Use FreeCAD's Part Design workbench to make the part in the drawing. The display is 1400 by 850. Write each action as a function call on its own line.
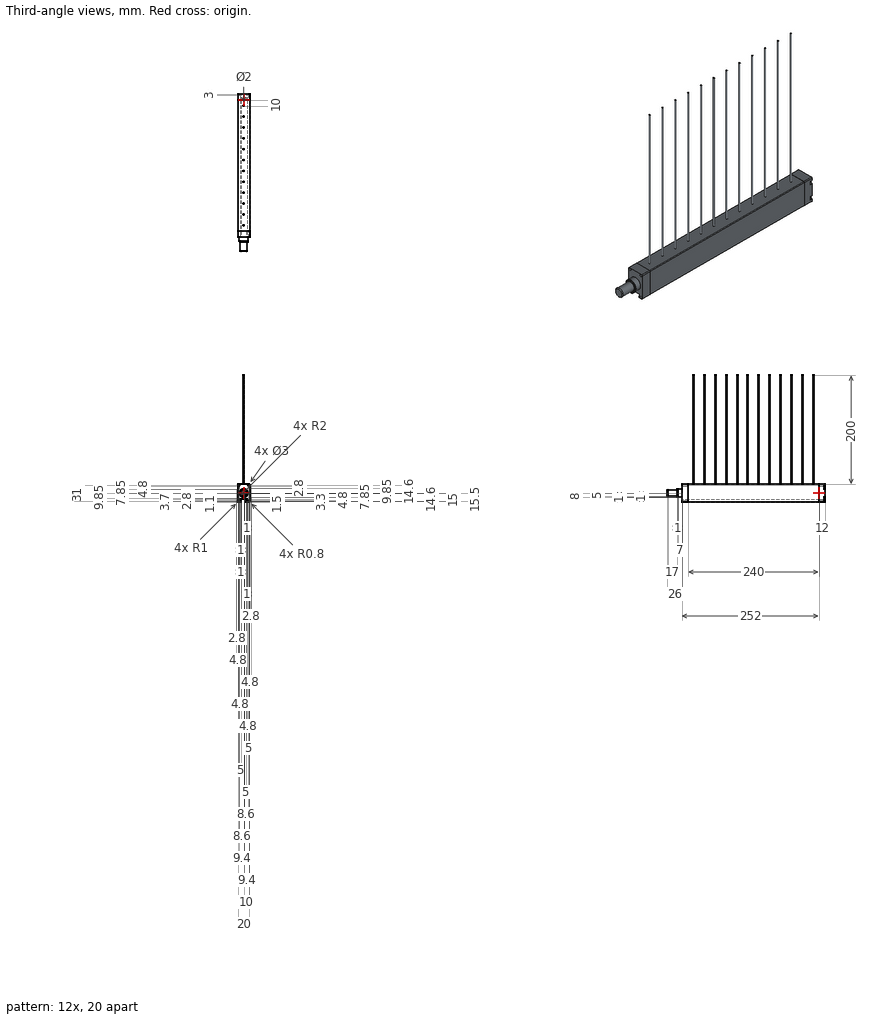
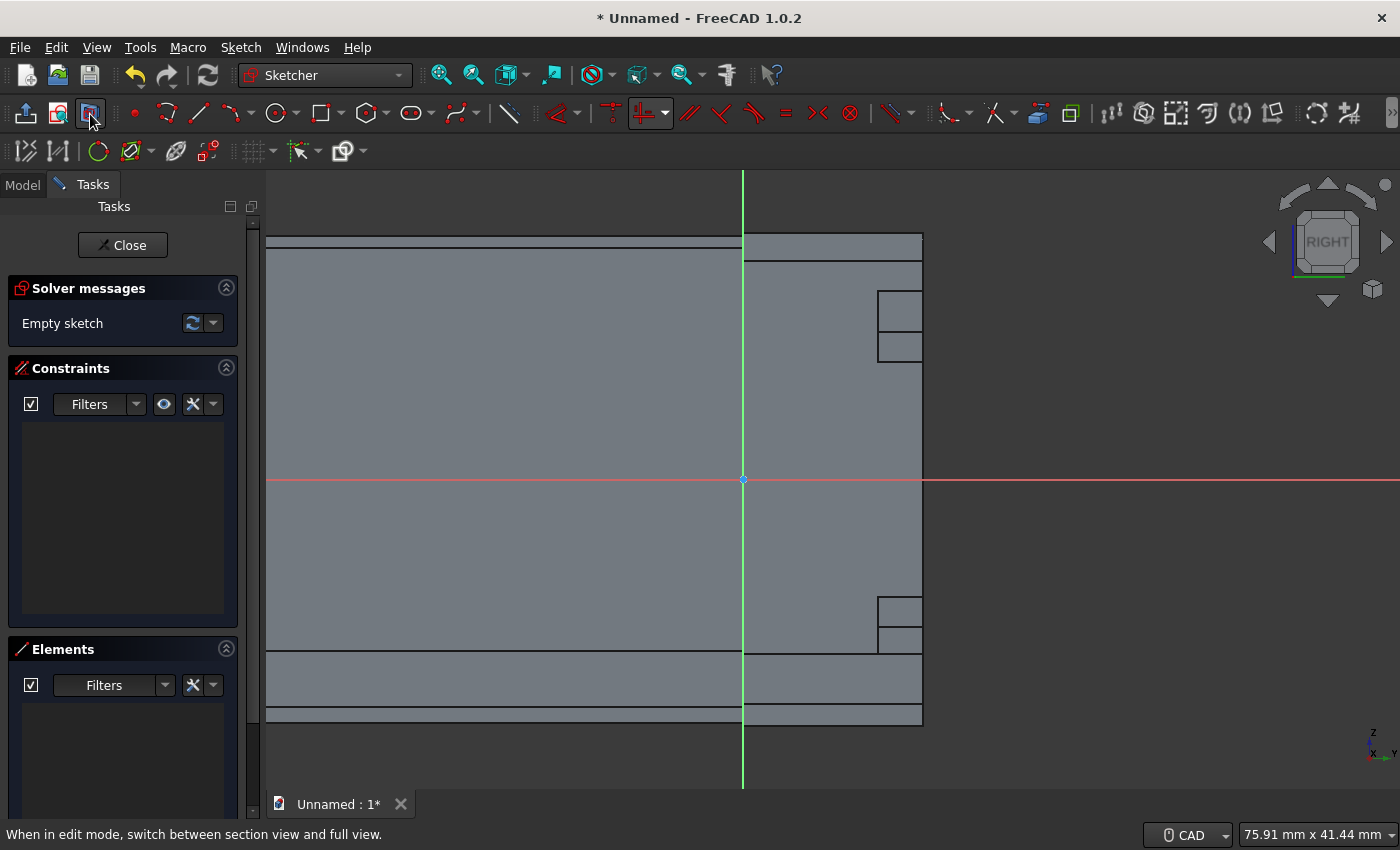
scroll(764, 480, down, 5)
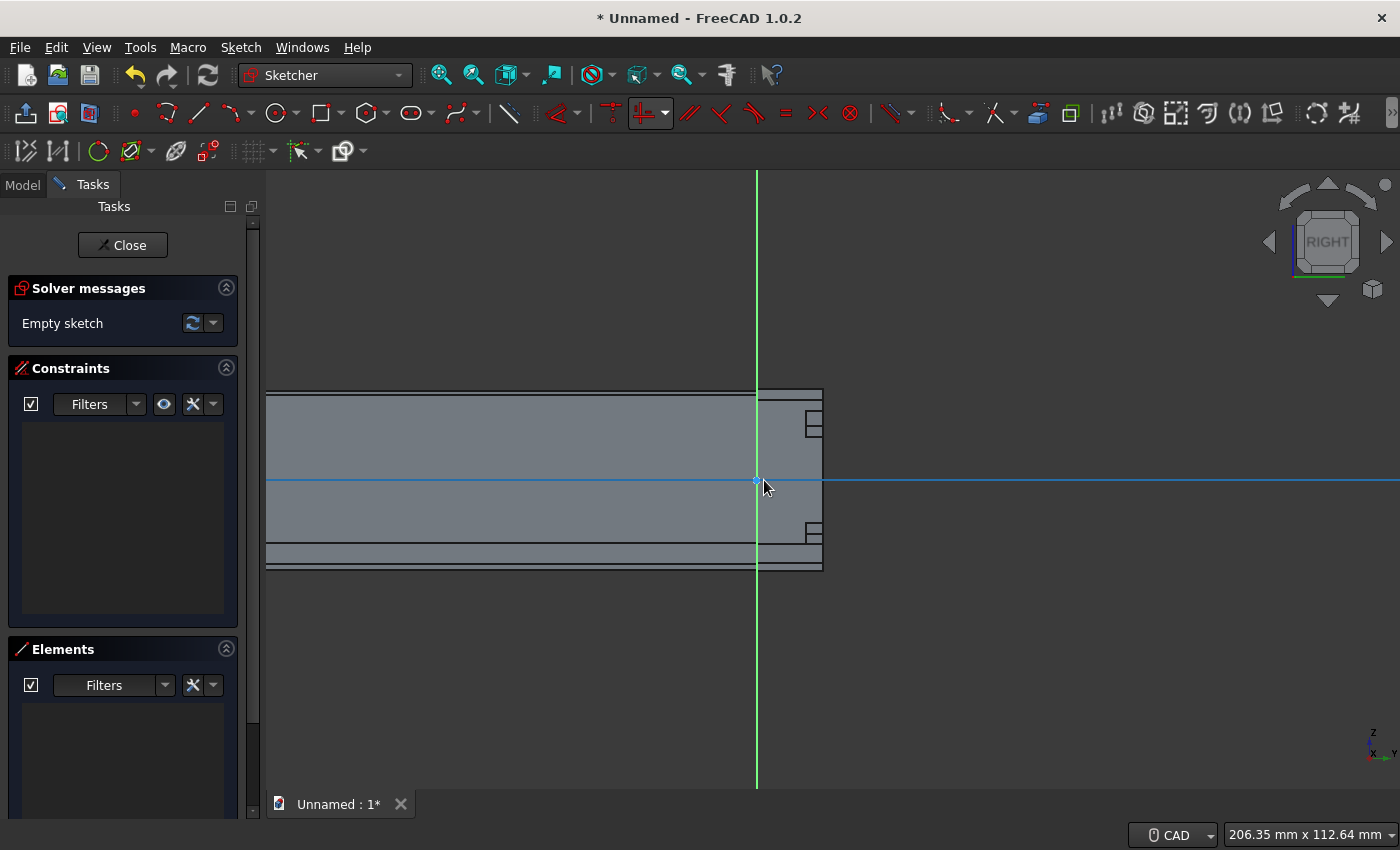
scroll(764, 480, down, 5)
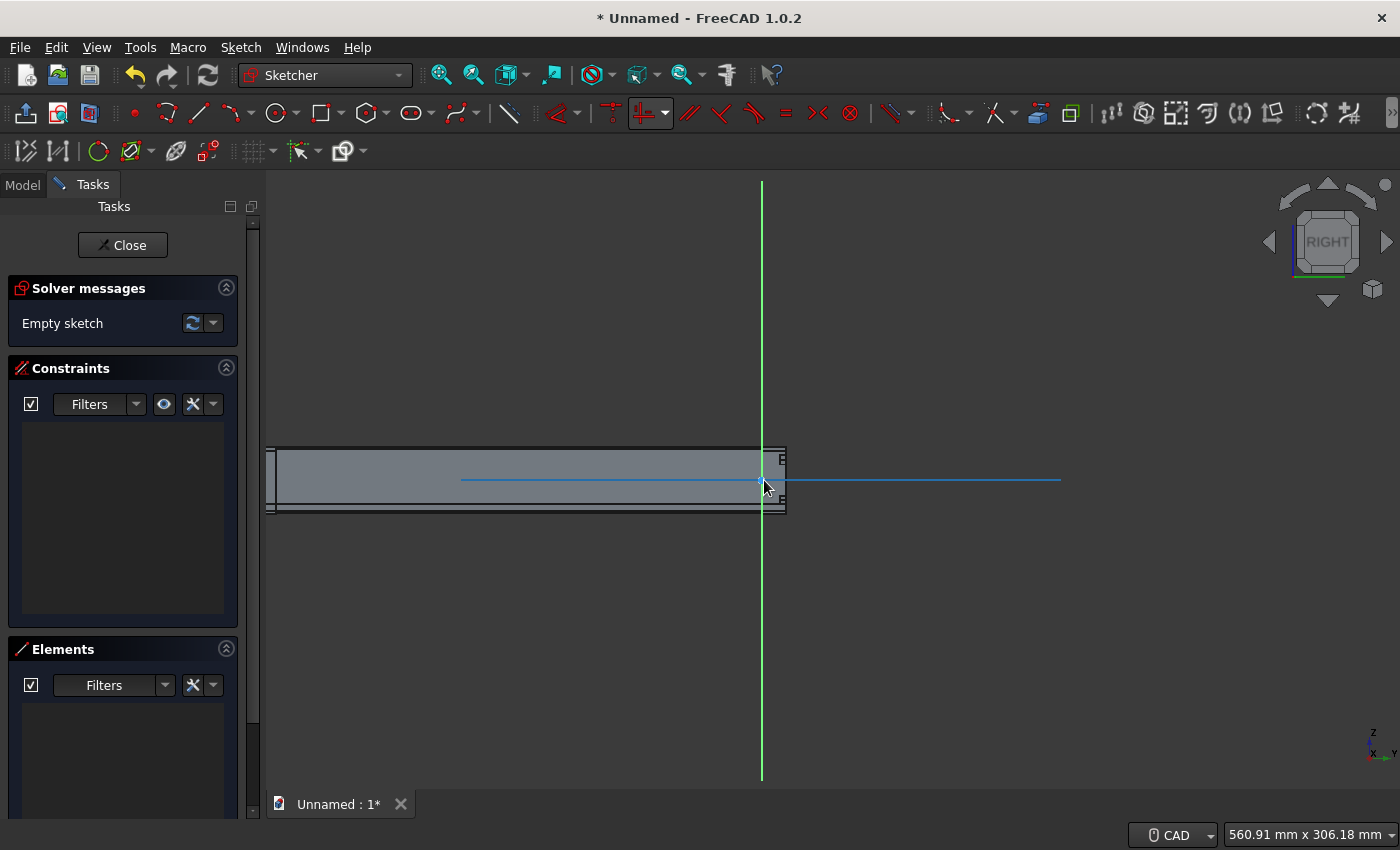
scroll(764, 480, down, 5)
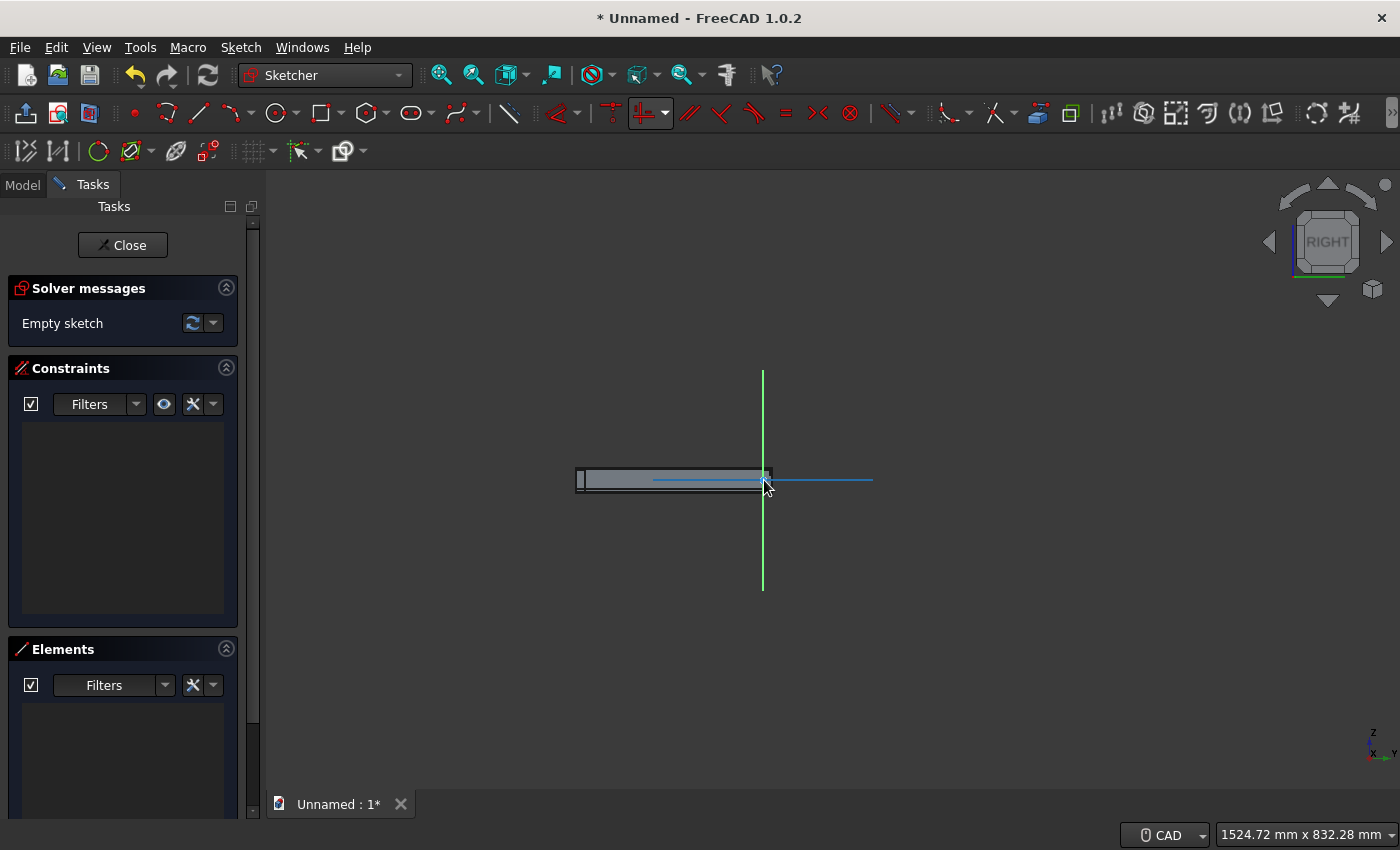
scroll(556, 484, up, 15)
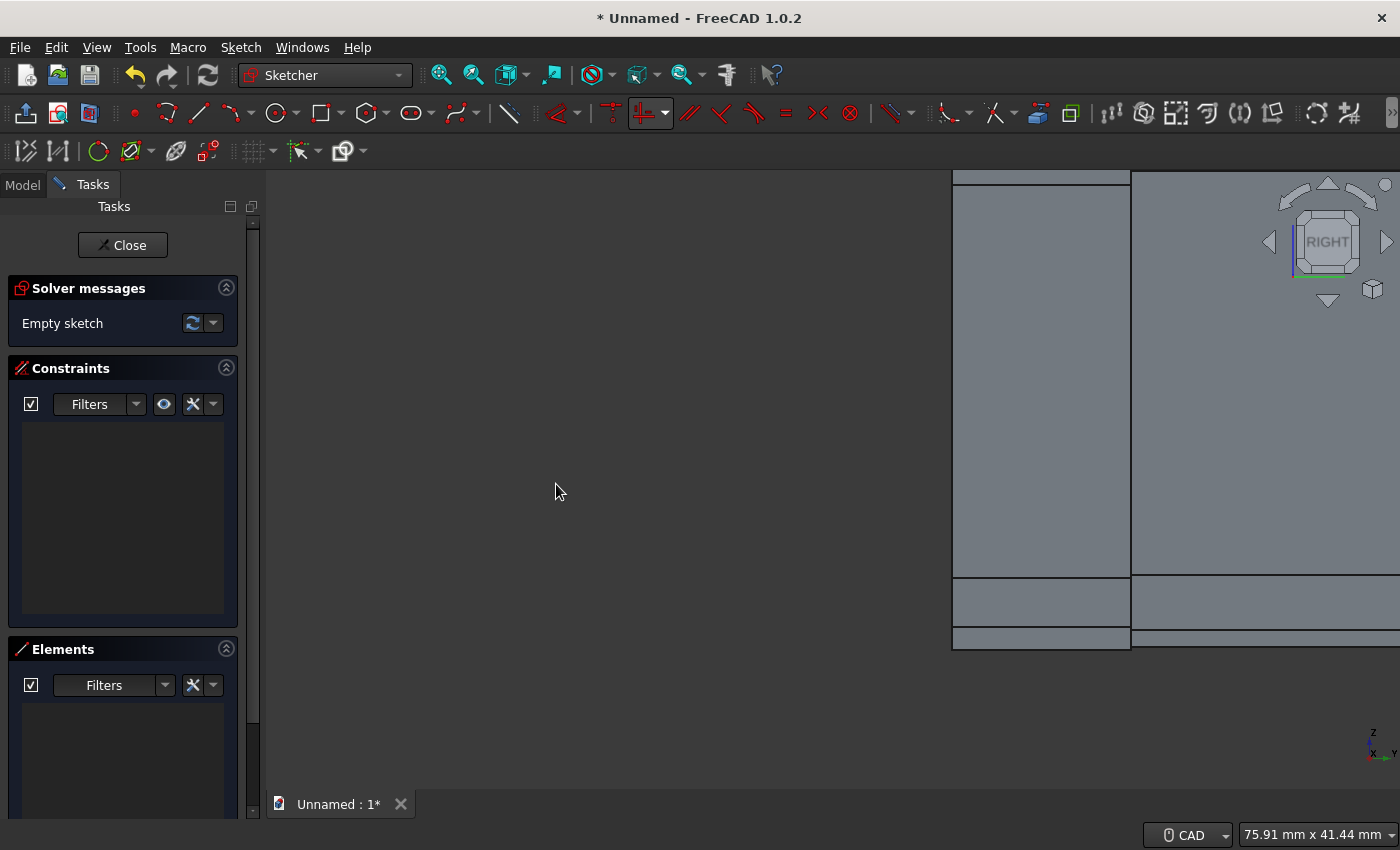
scroll(750, 442, up, 3)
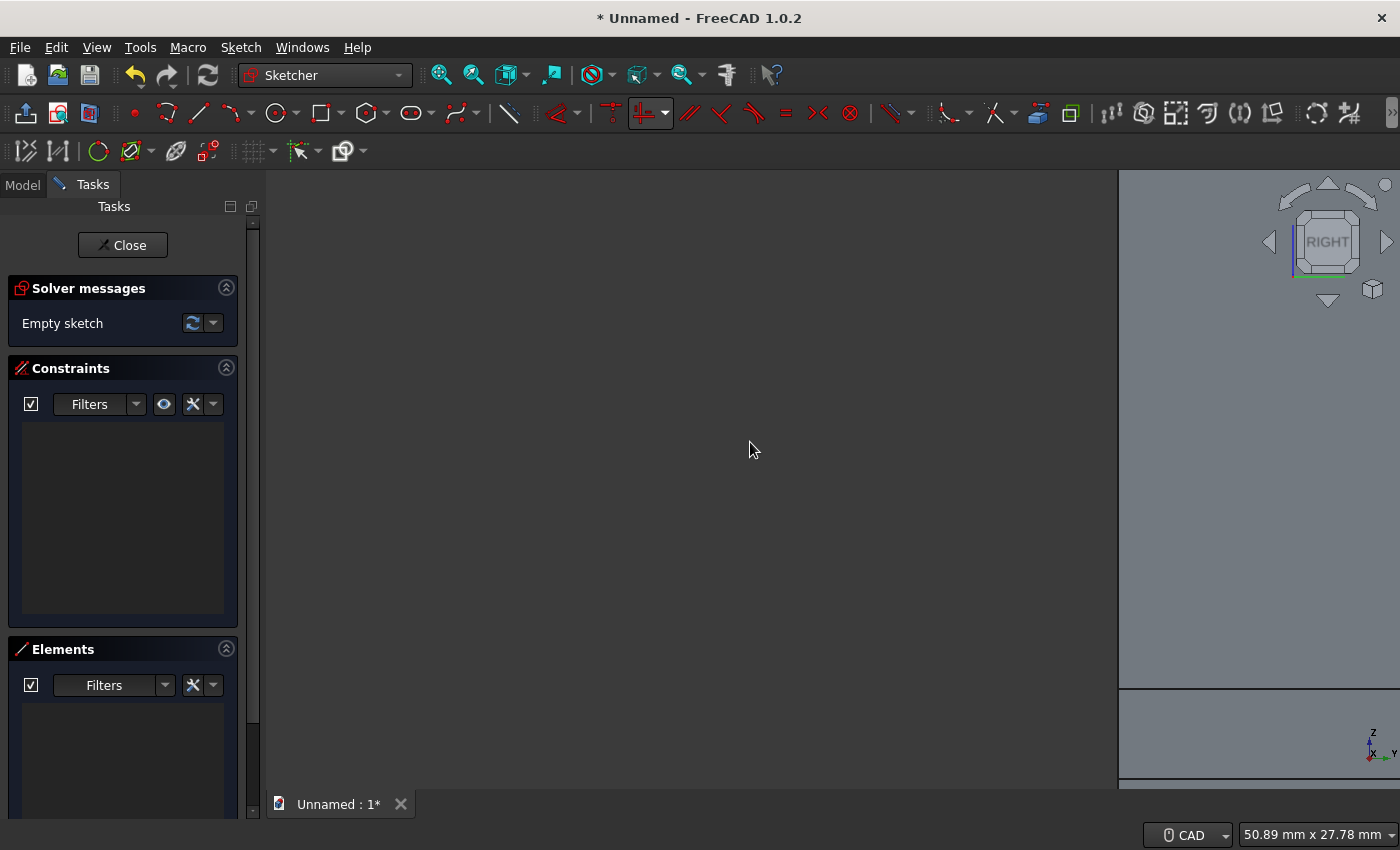
click(168, 114)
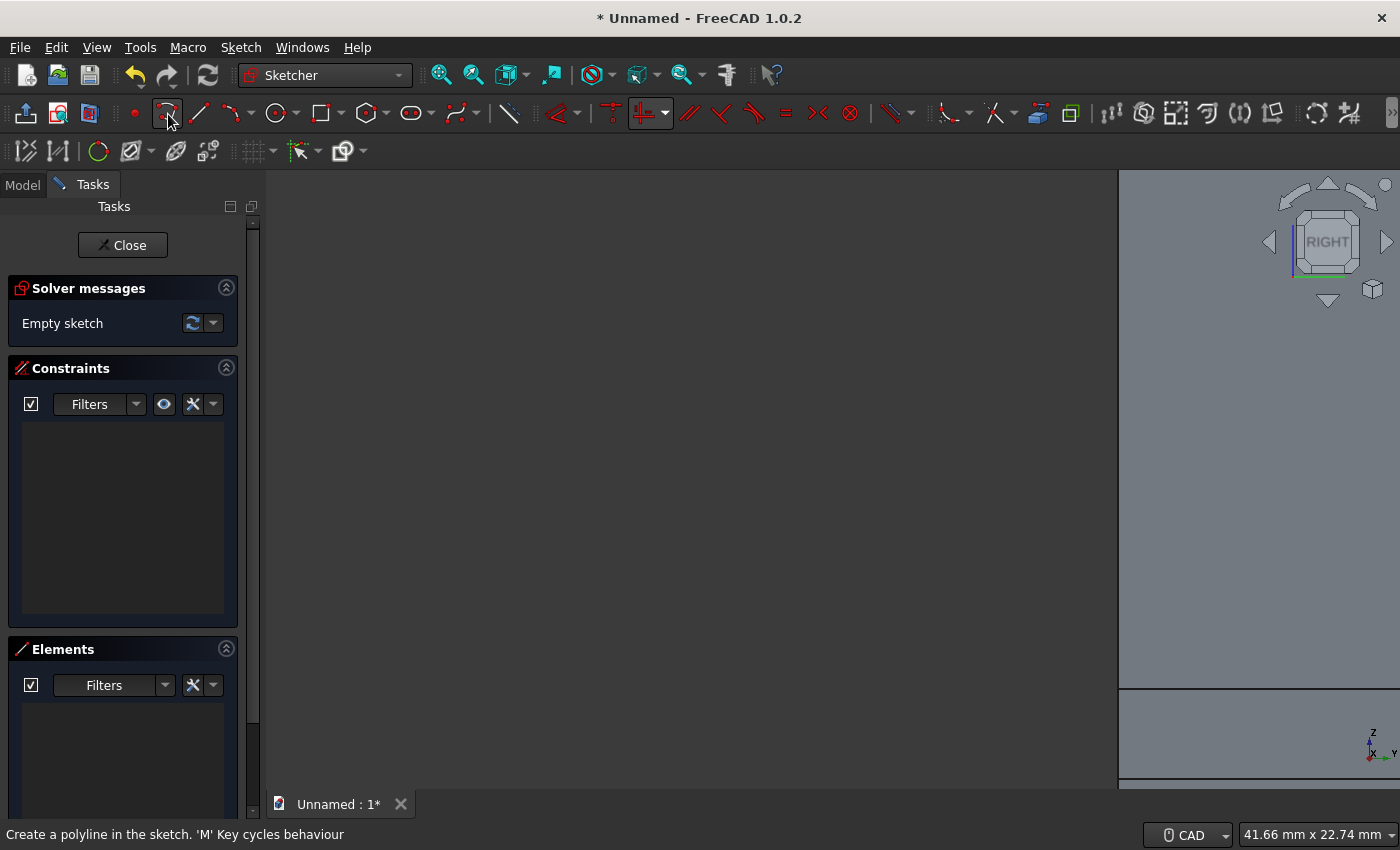
click(1118, 371)
click(410, 380)
click(410, 507)
click(438, 534)
click(900, 534)
click(900, 561)
click(928, 561)
click(928, 588)
click(1118, 588)
click(1118, 372)
key(Escape)
key(Escape)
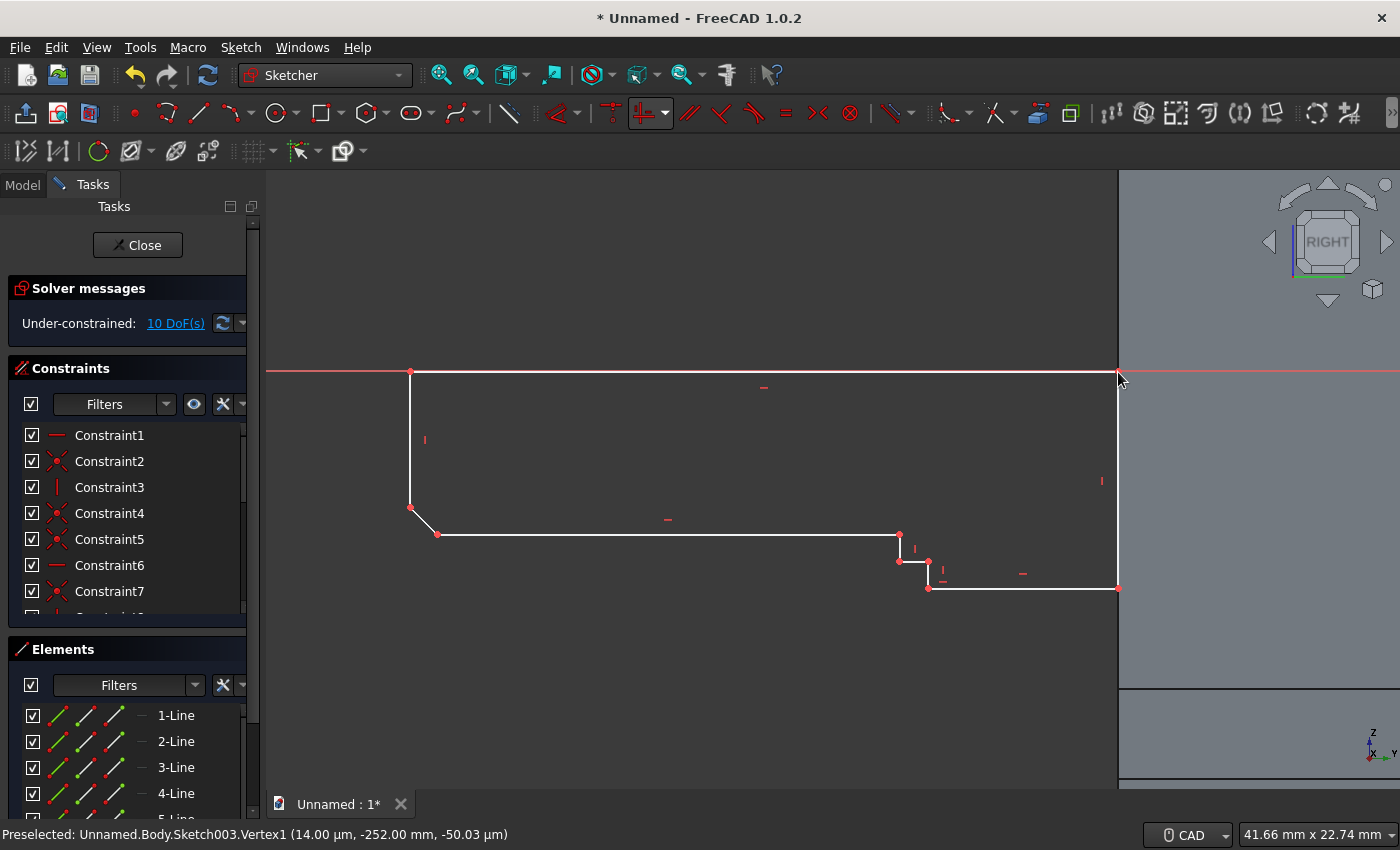
click(1118, 372)